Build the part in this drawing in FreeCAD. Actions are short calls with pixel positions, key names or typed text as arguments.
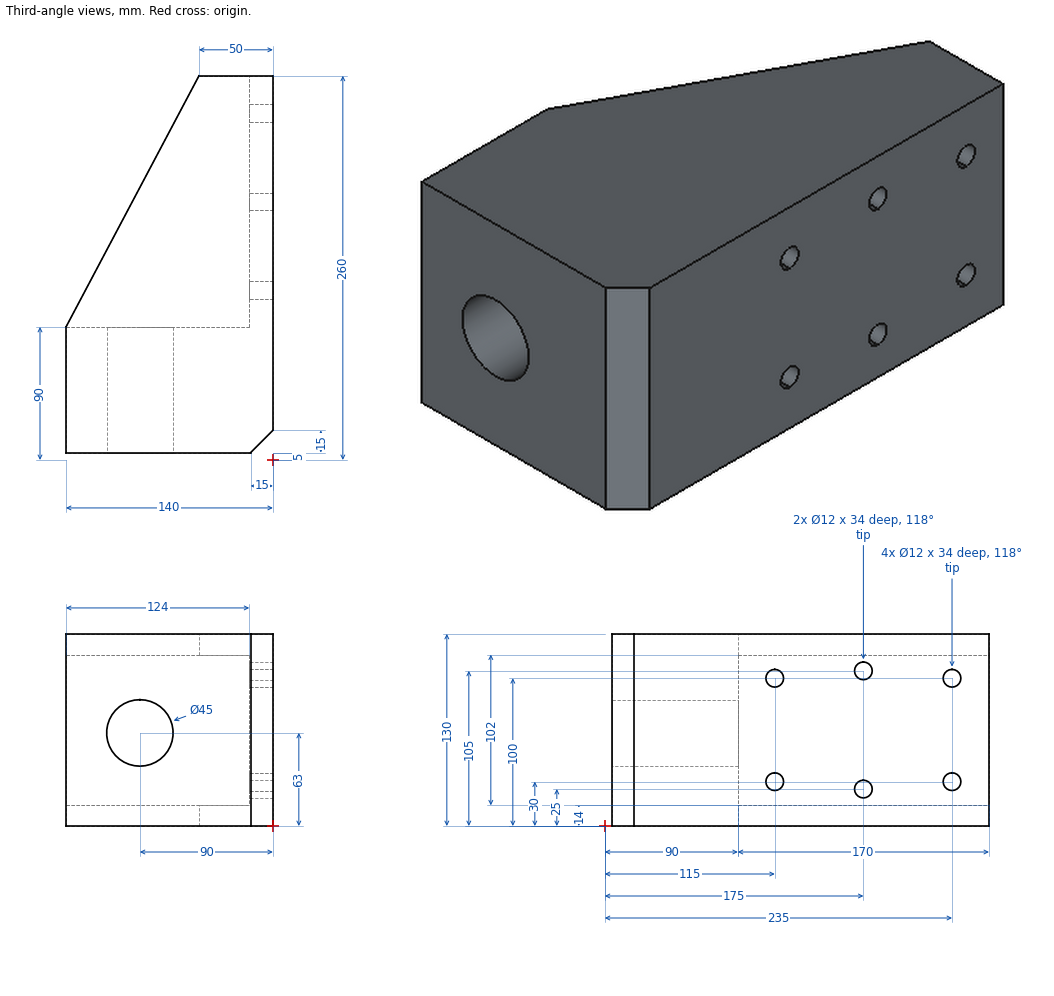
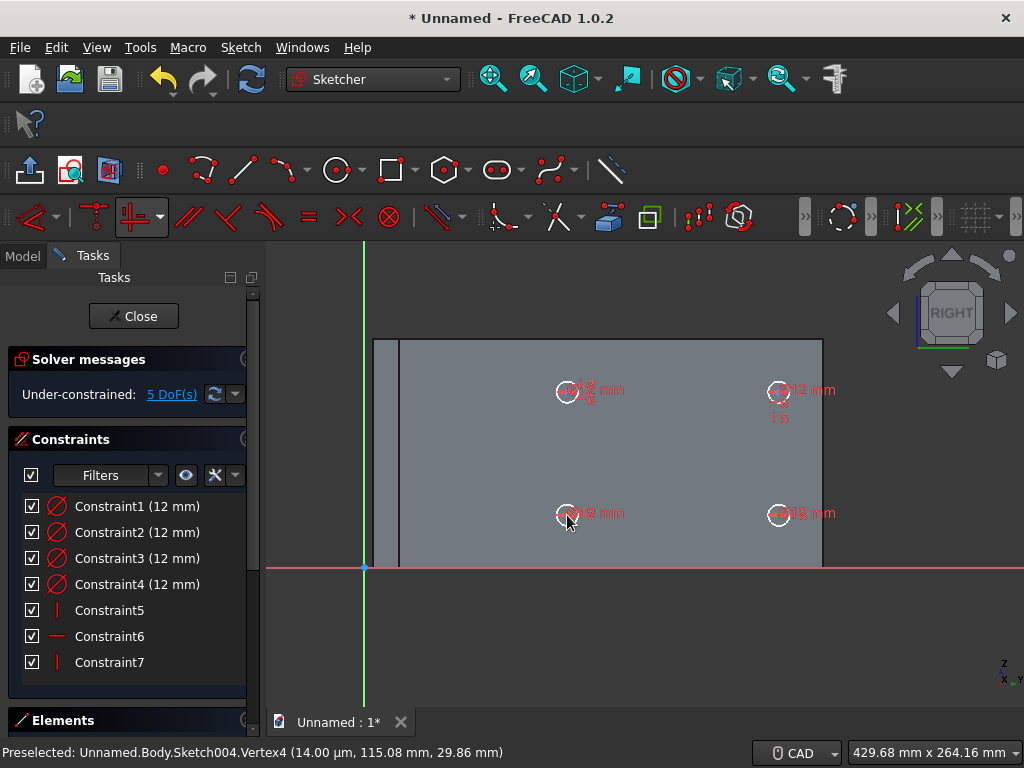
key(h)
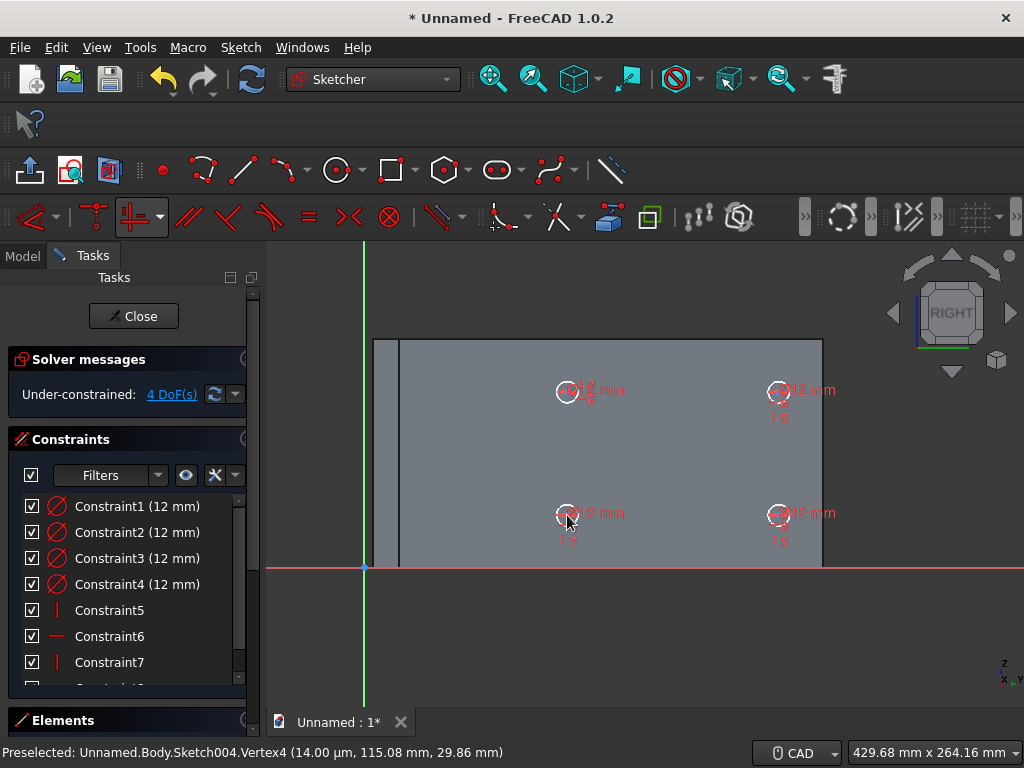
click(32, 218)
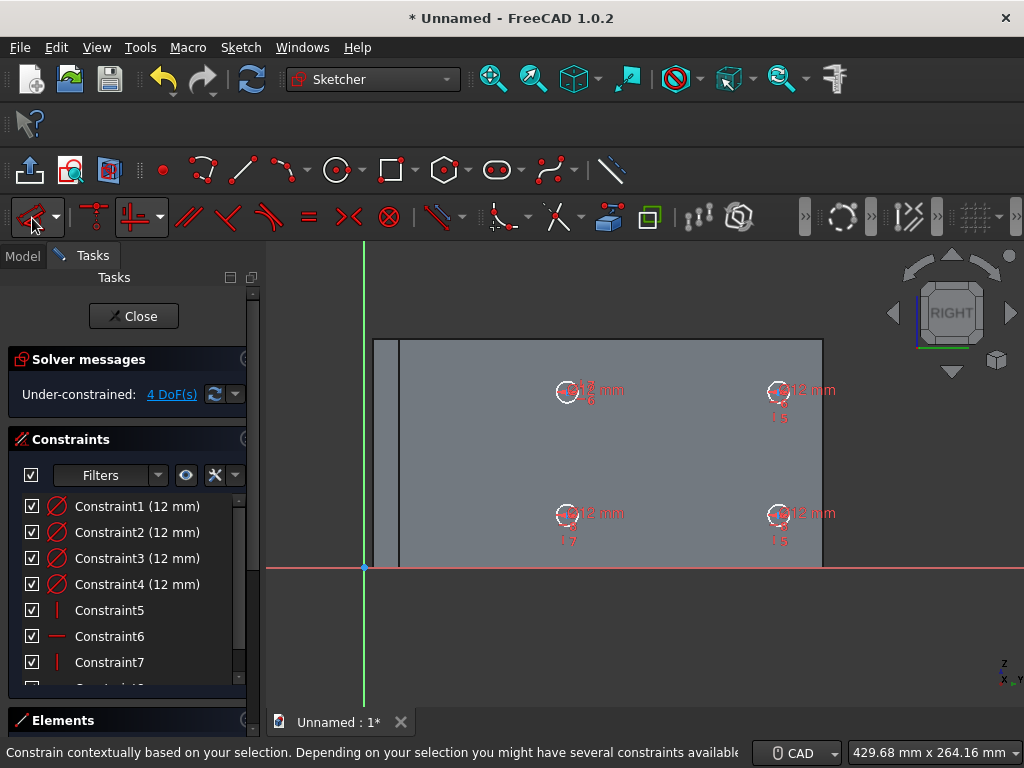
click(779, 515)
click(330, 542)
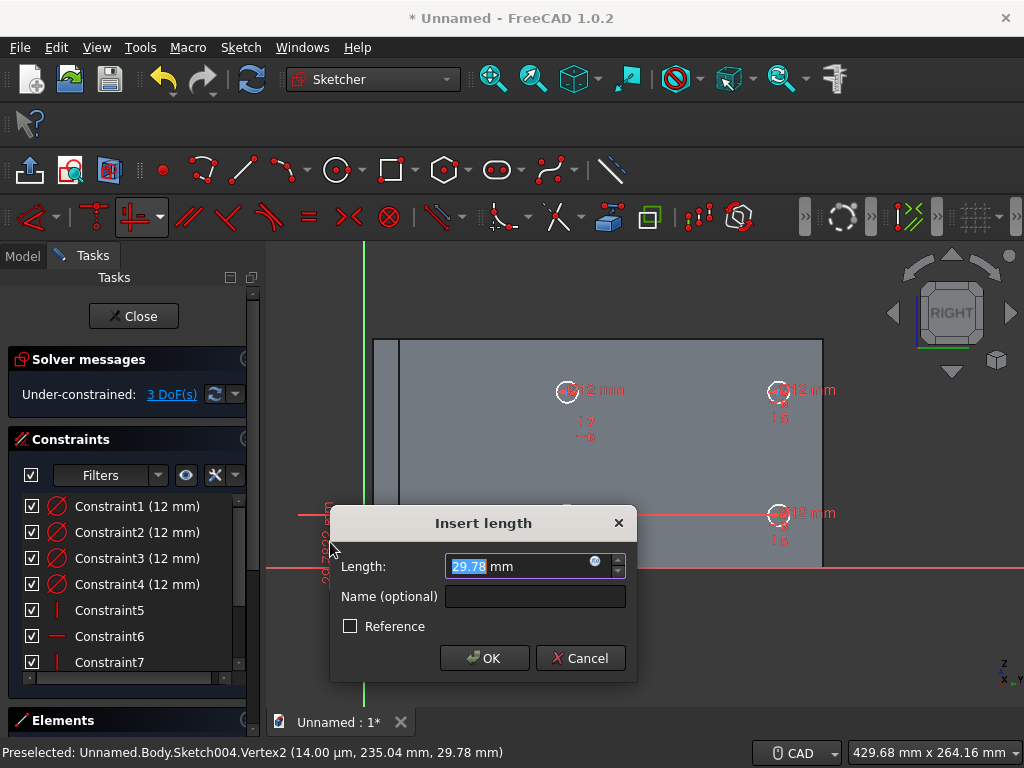
text(30)
key(Return)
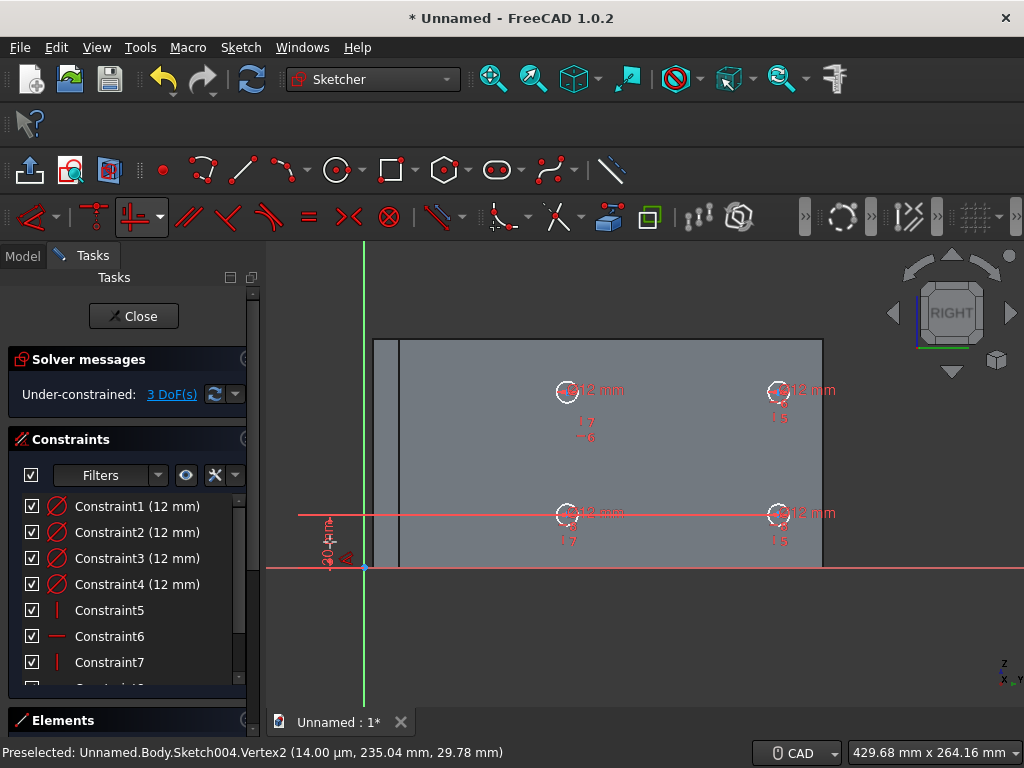
click(779, 392)
click(572, 602)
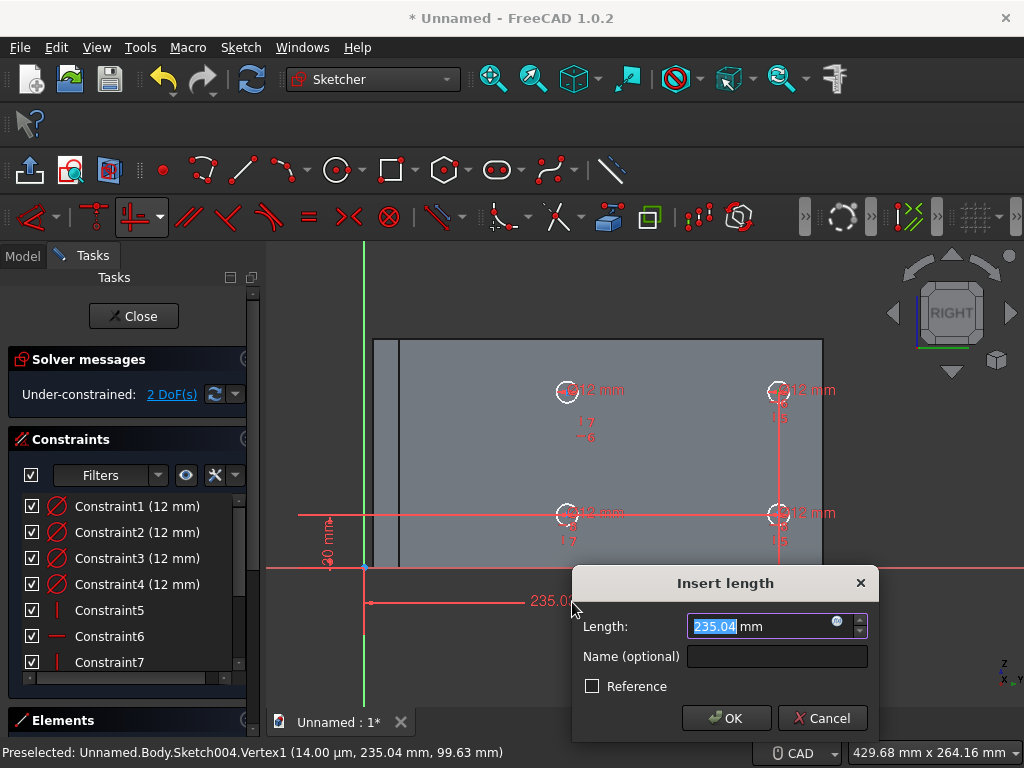
text(235)
key(Return)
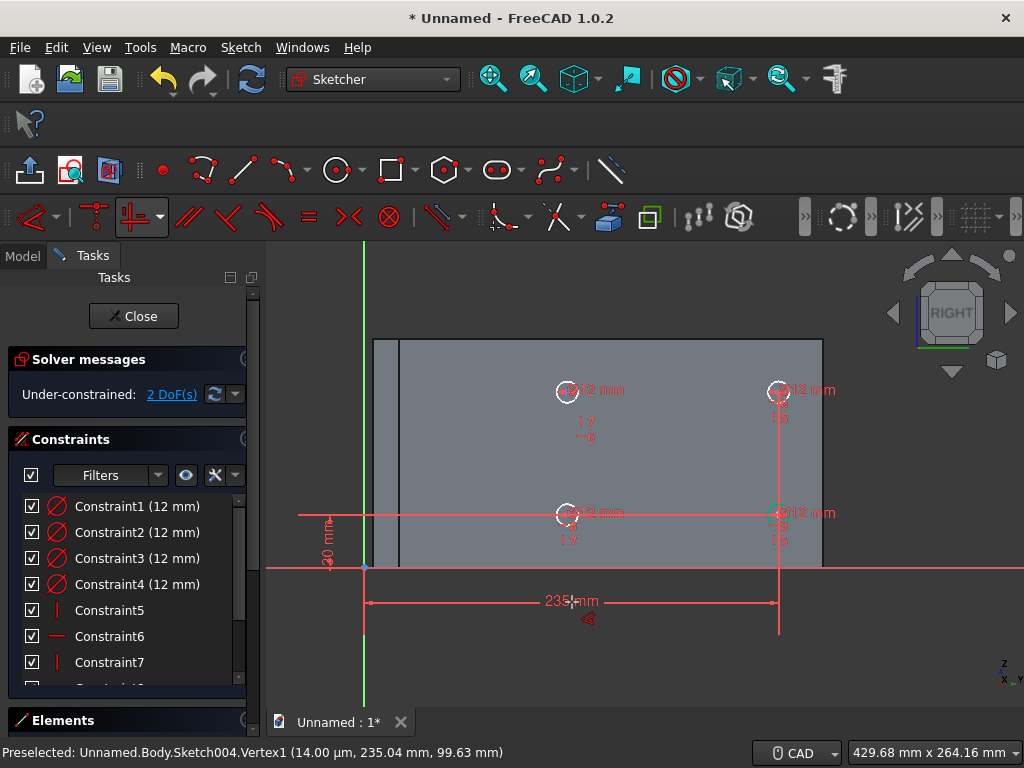
click(779, 392)
click(330, 480)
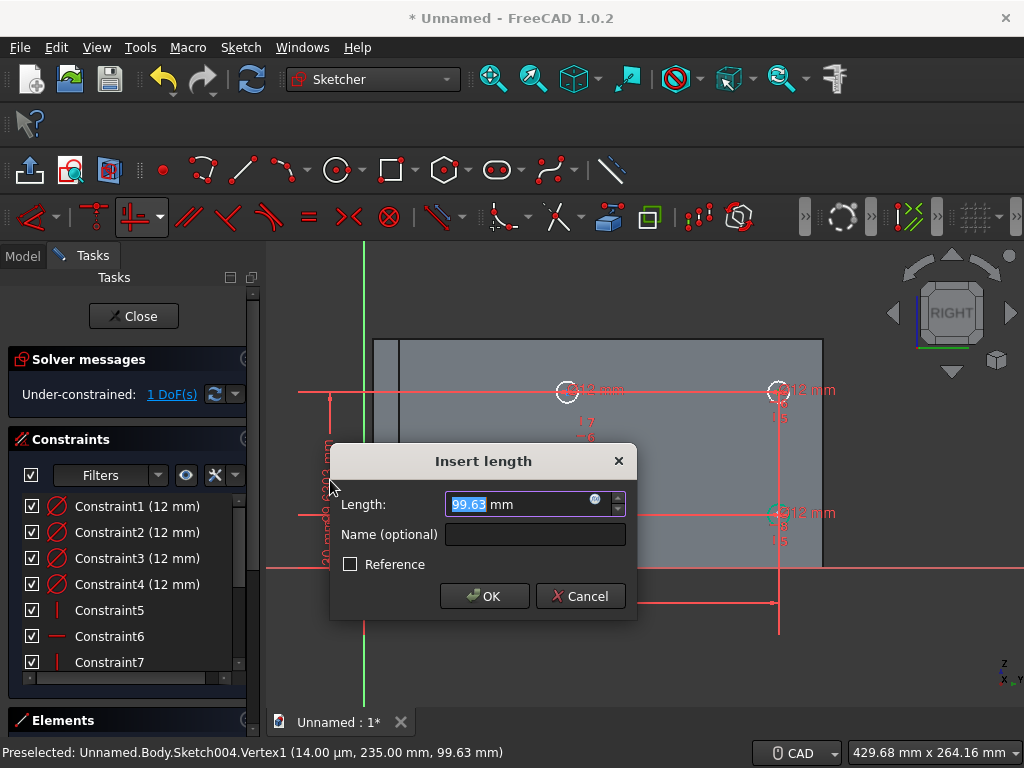
text(100)
key(Return)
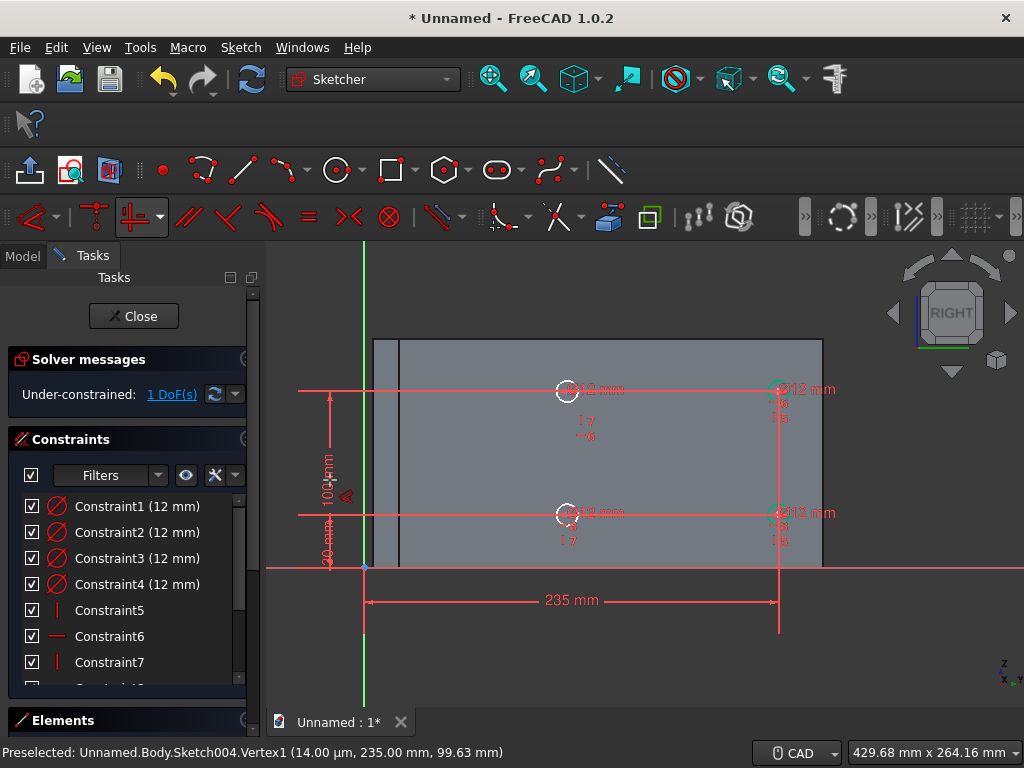
click(567, 391)
click(466, 602)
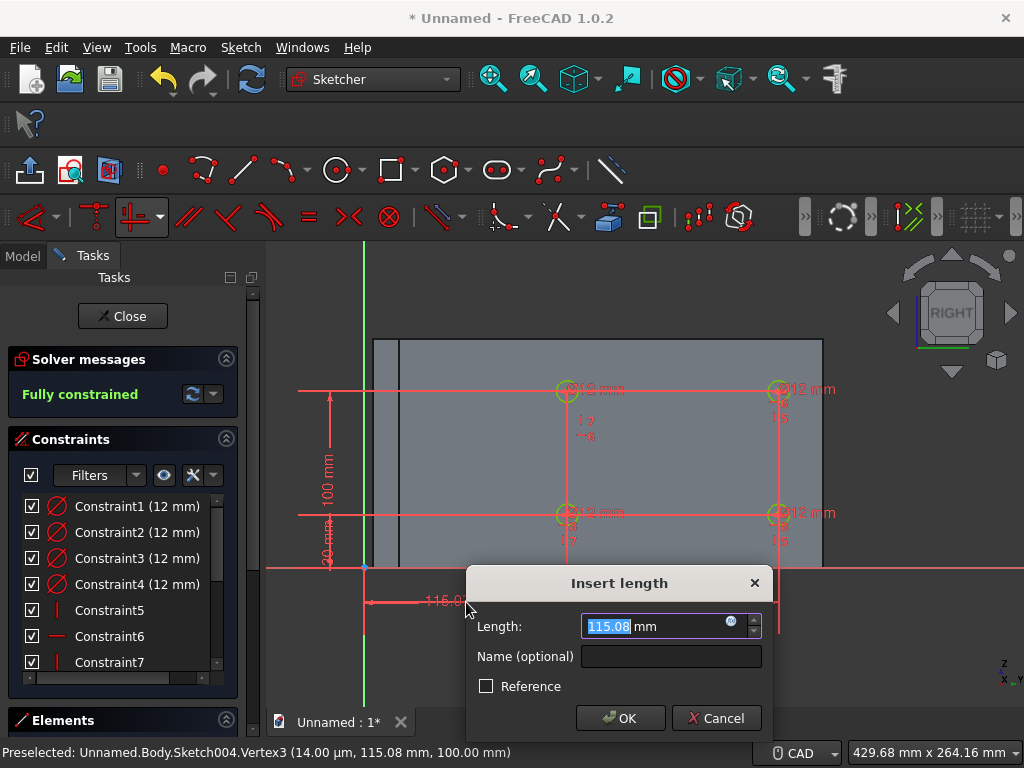
text(115)
key(Return)
key(Escape)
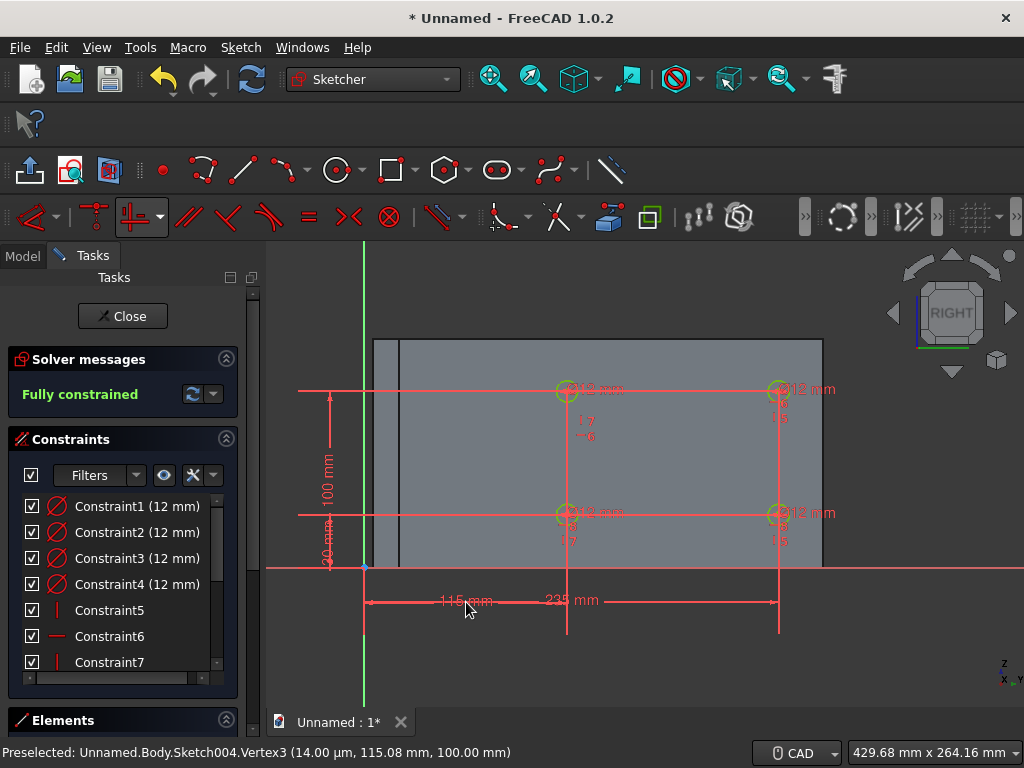
click(123, 316)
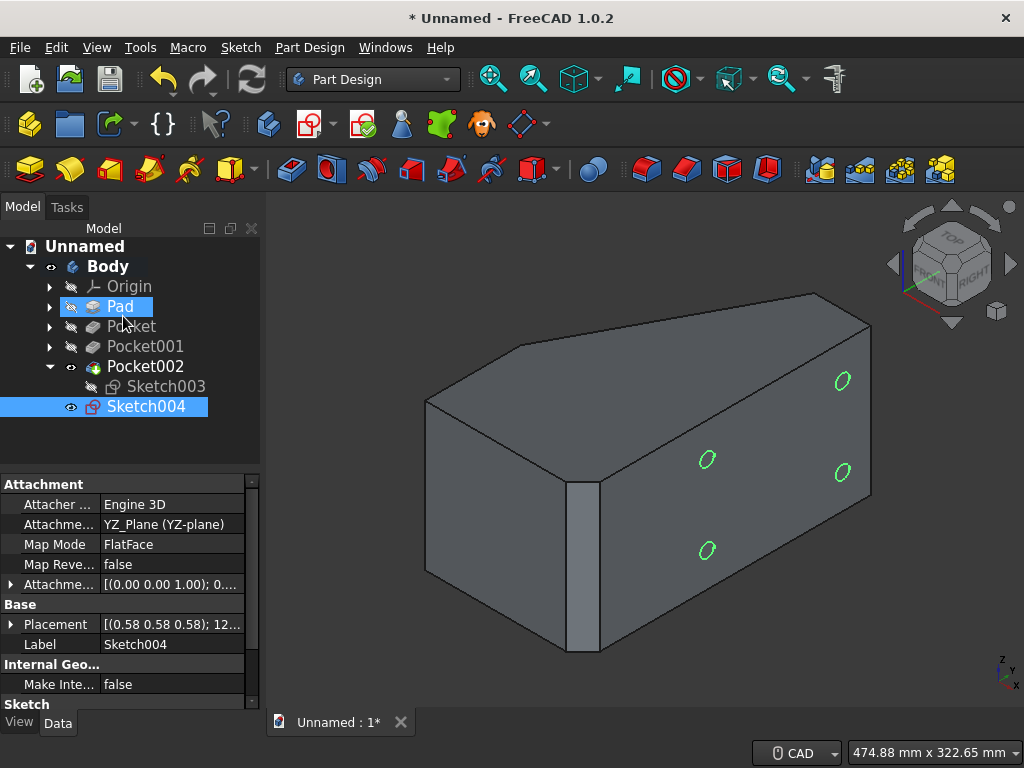
click(332, 170)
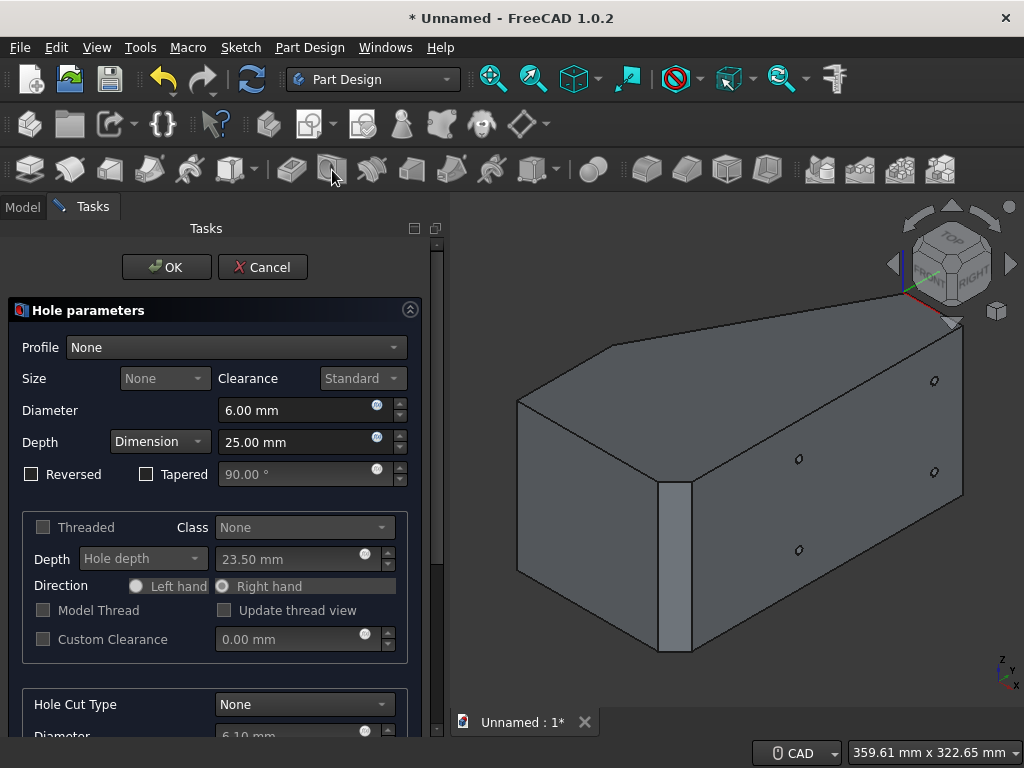
triple_click(305, 410)